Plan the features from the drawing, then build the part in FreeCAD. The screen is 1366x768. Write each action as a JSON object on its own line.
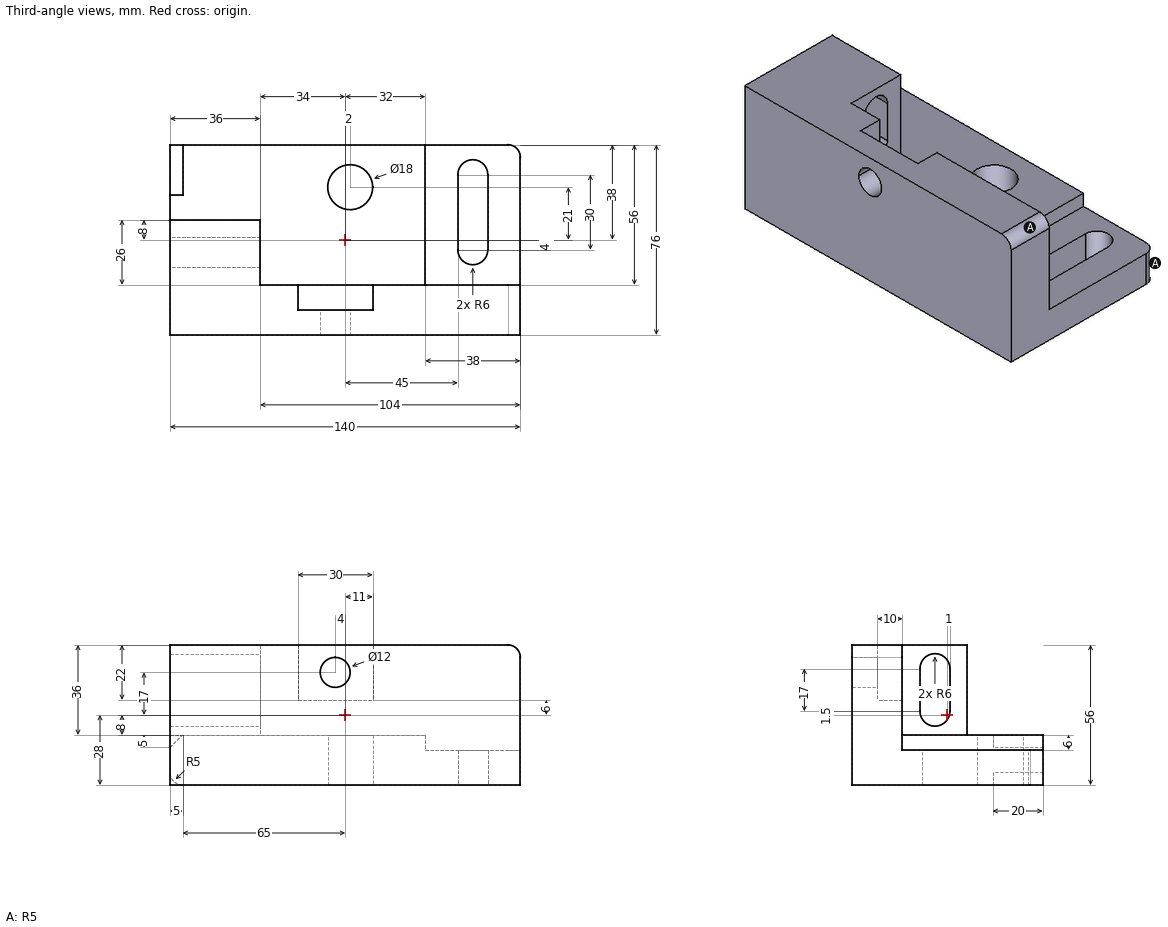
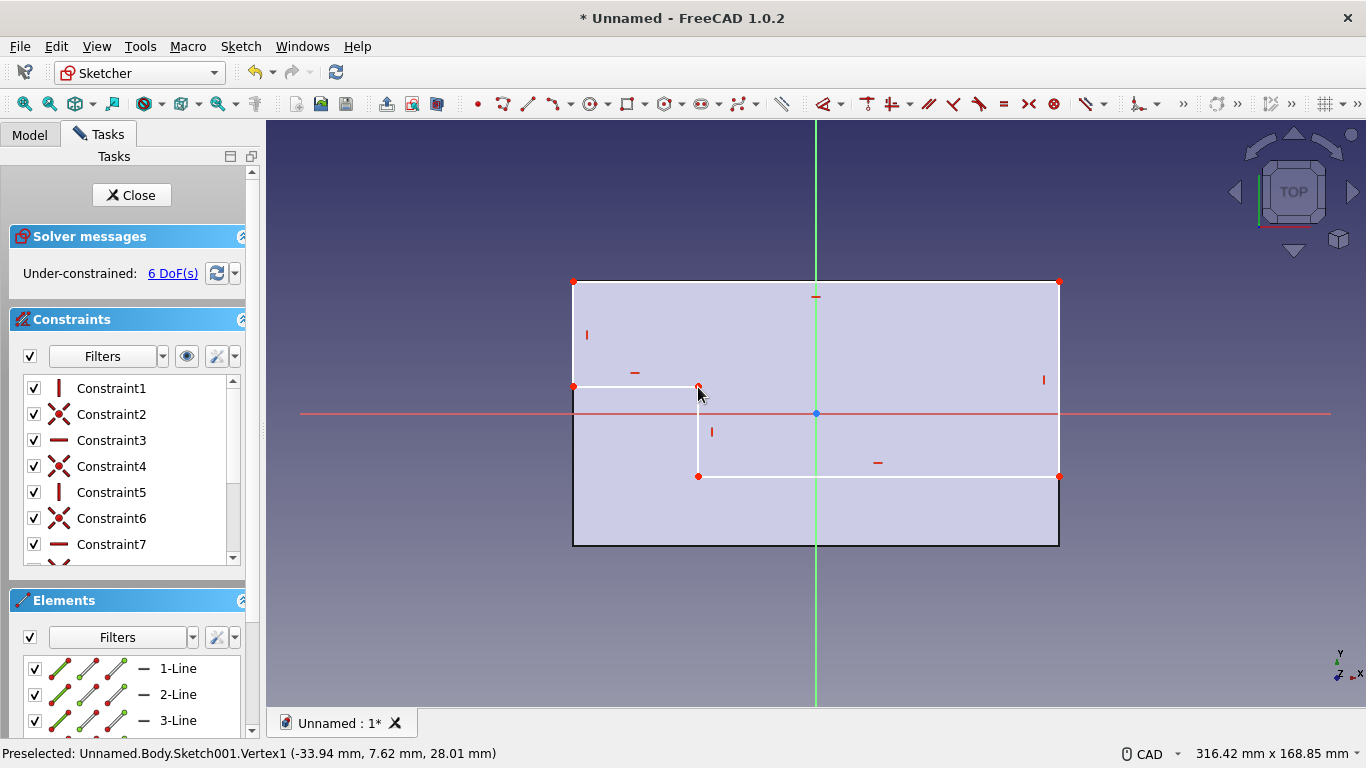
{"action": "left_click", "coordinate": [698, 414]}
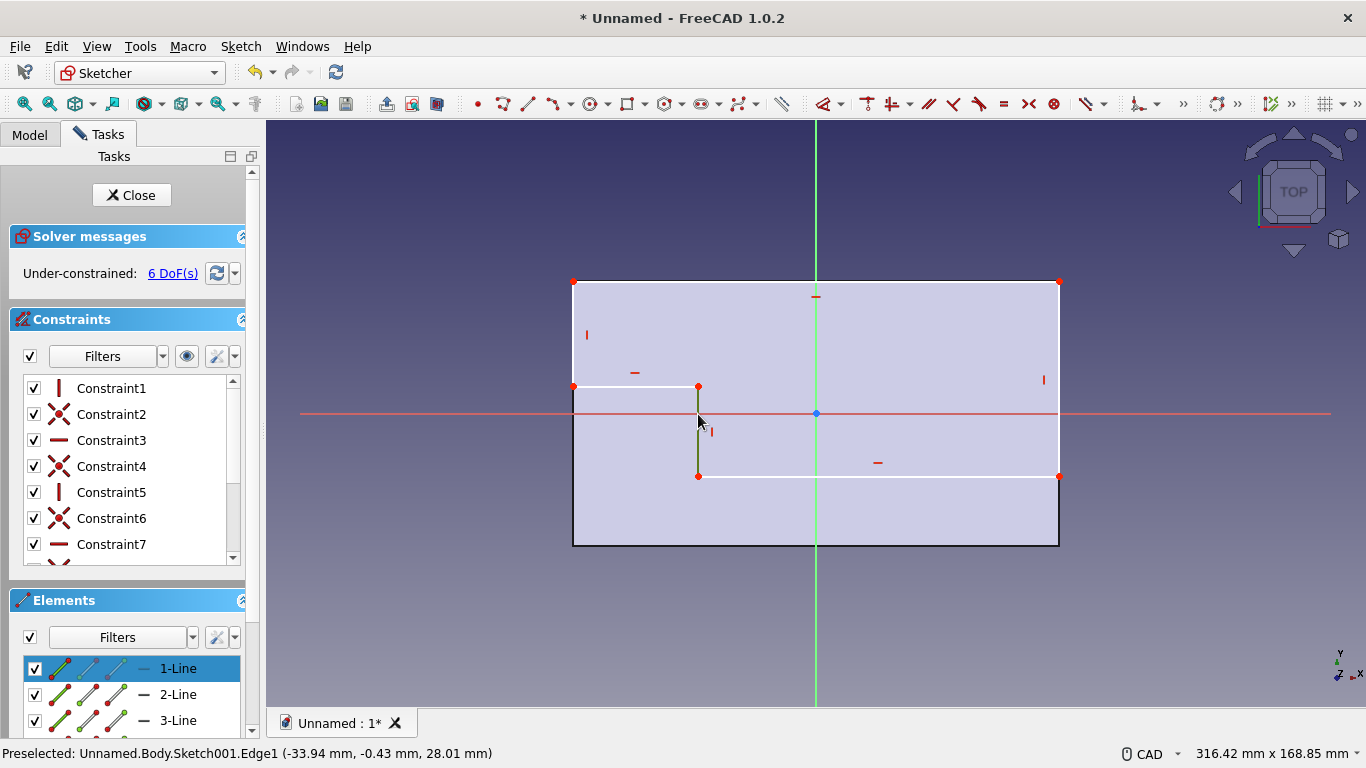
{"action": "key", "text": "i"}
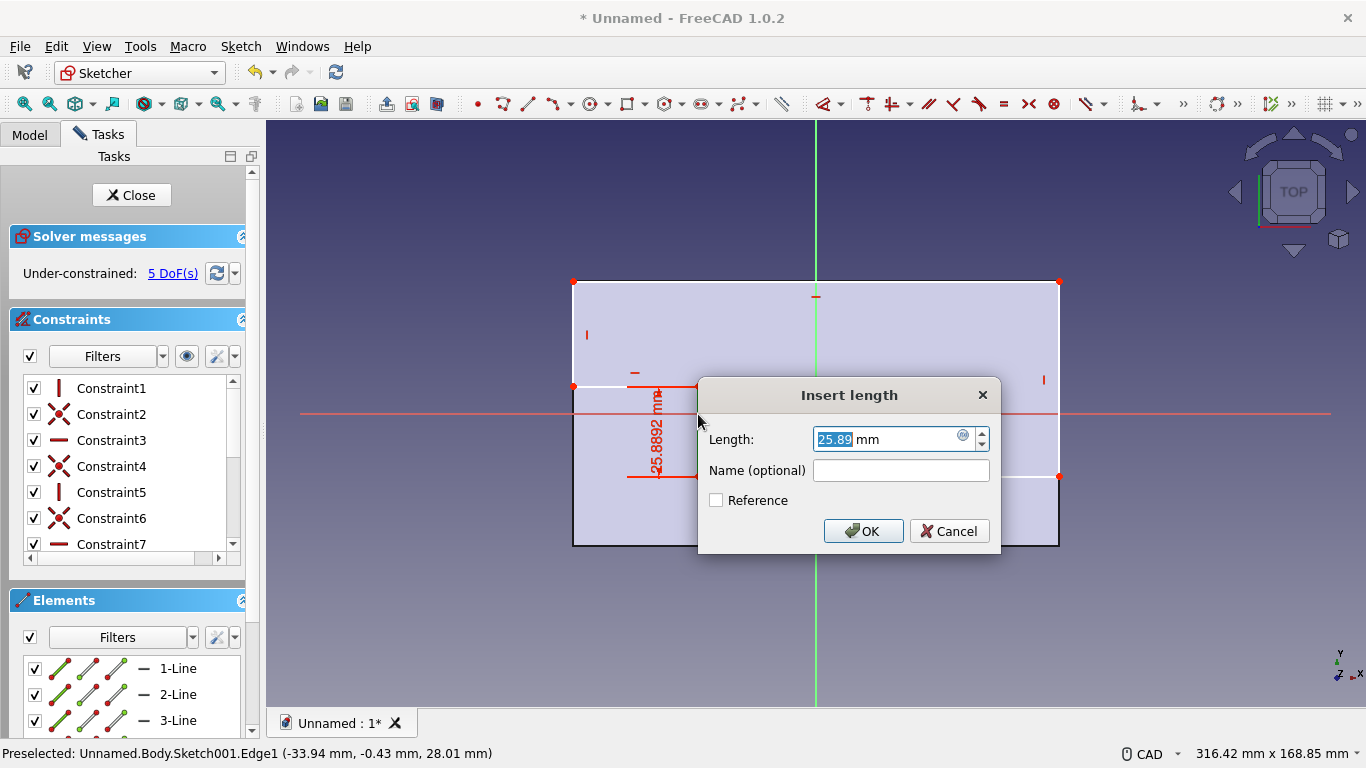
{"action": "type", "text": "26"}
{"action": "key", "text": "Return"}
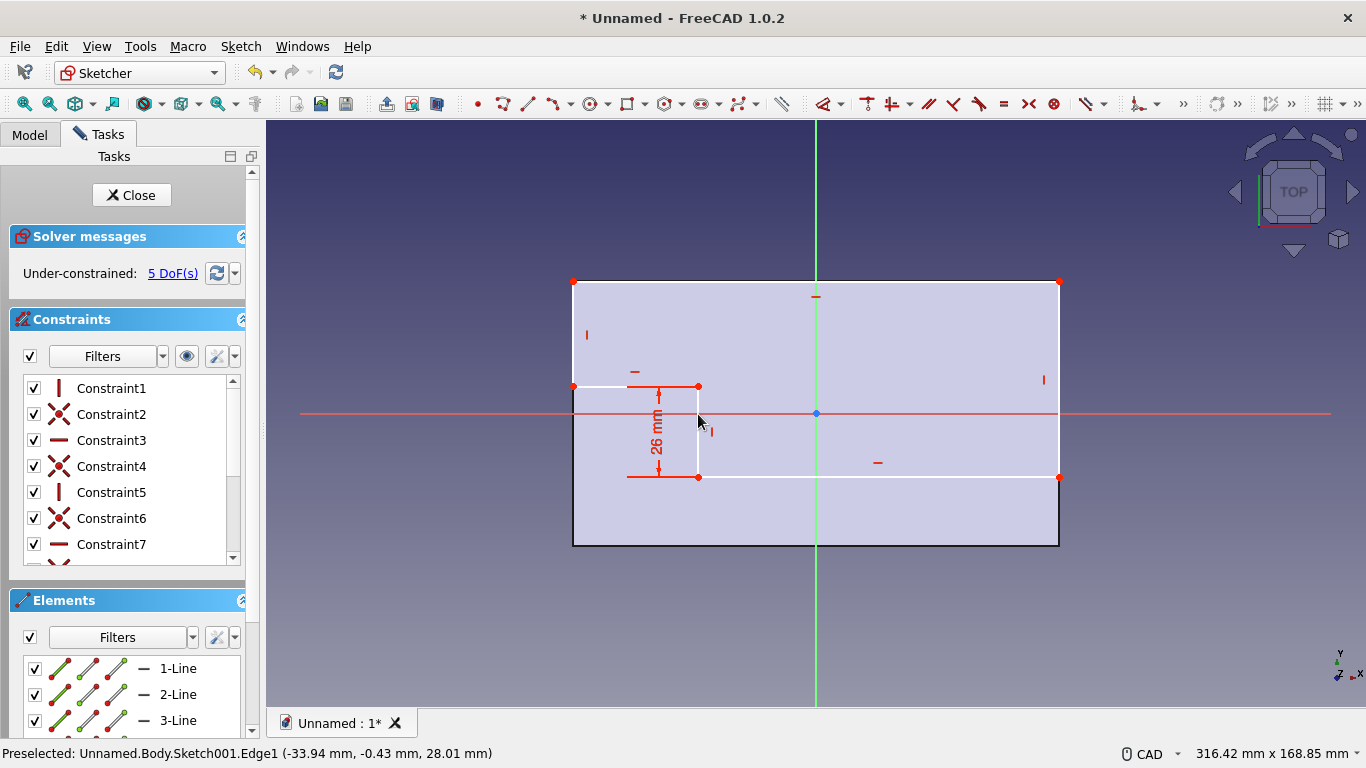
{"action": "left_click", "coordinate": [1059, 341]}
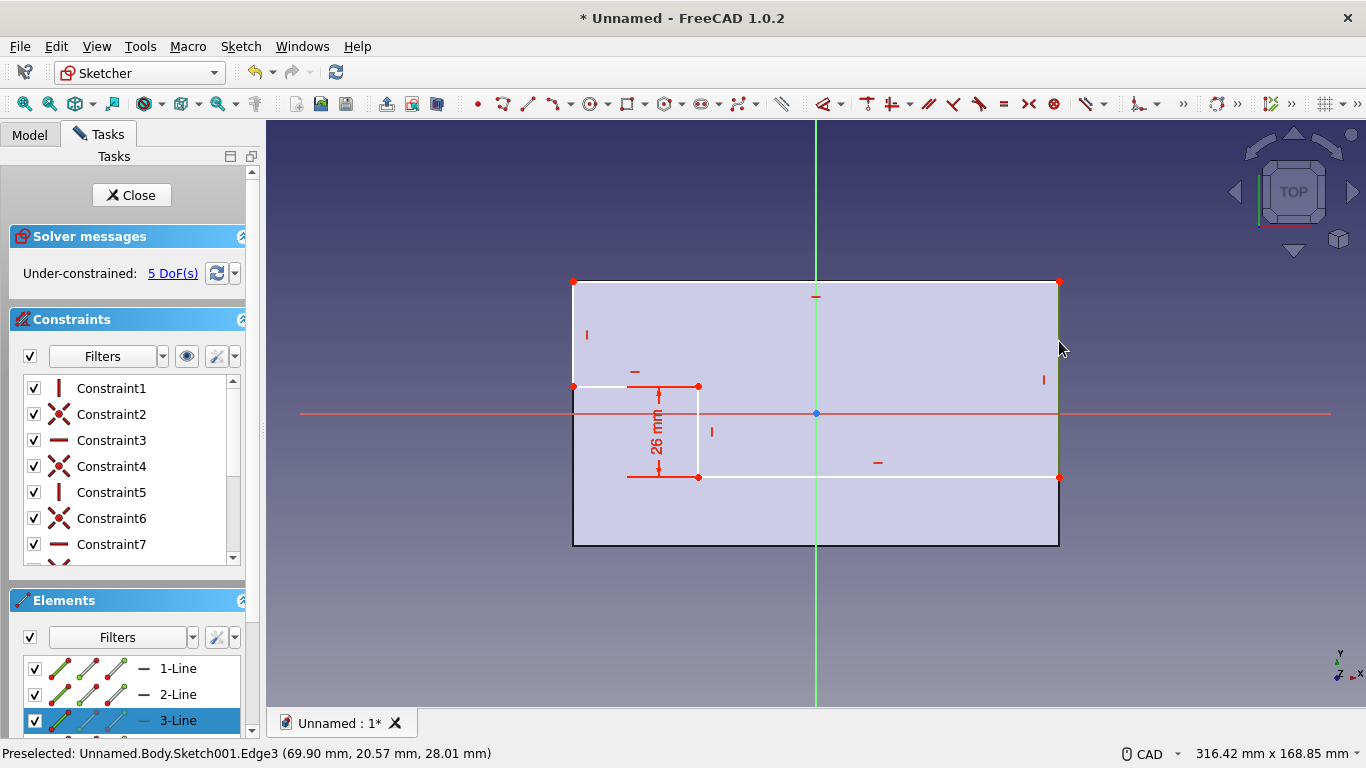
{"action": "left_click", "coordinate": [840, 104]}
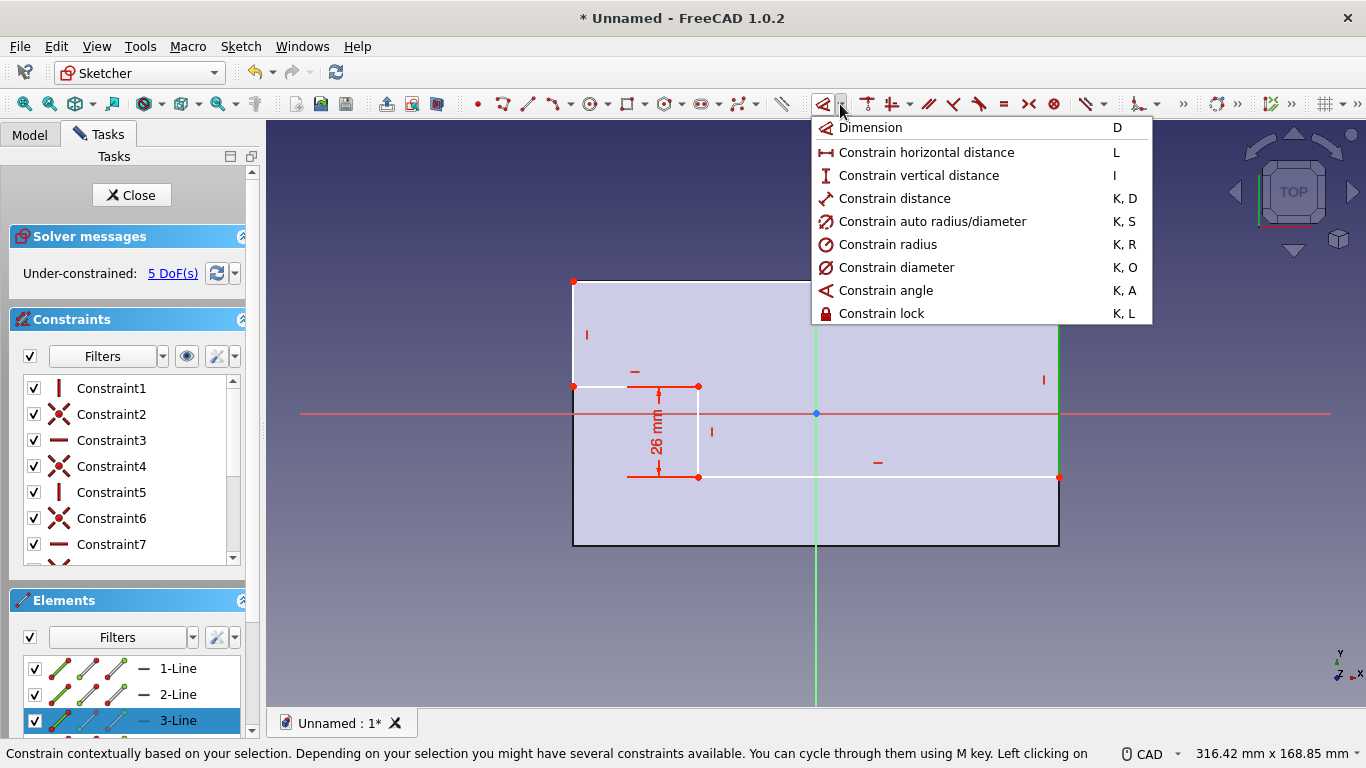
{"action": "left_click", "coordinate": [982, 176]}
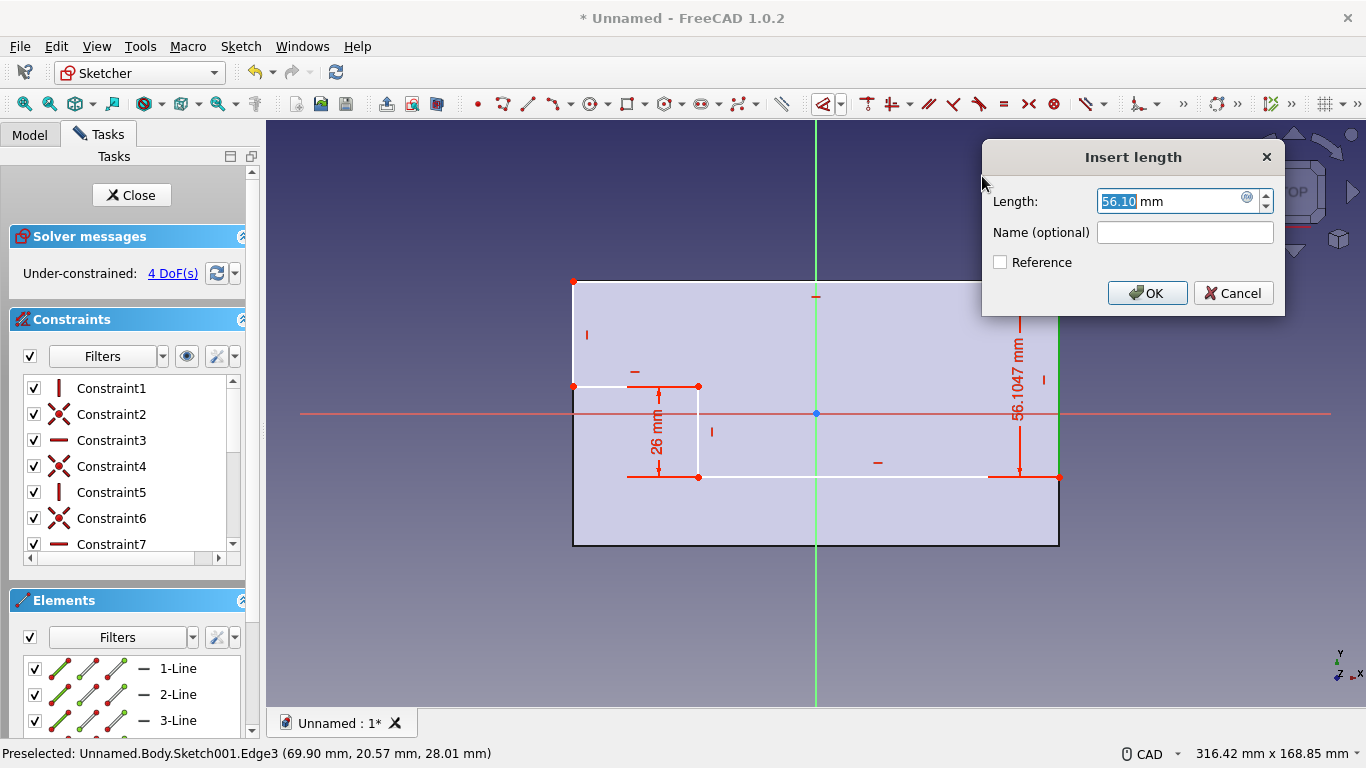
{"action": "type", "text": "56"}
{"action": "key", "text": "Return"}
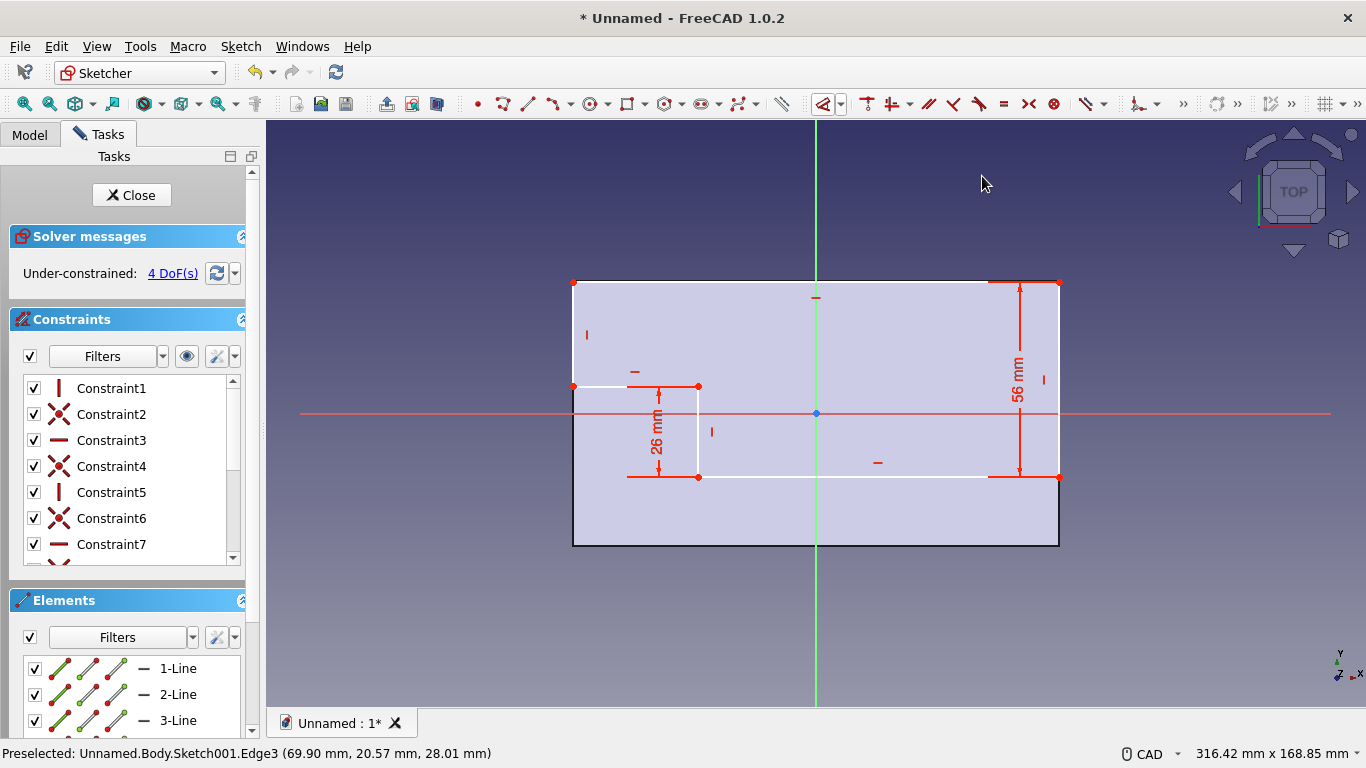
{"action": "left_click", "coordinate": [611, 387]}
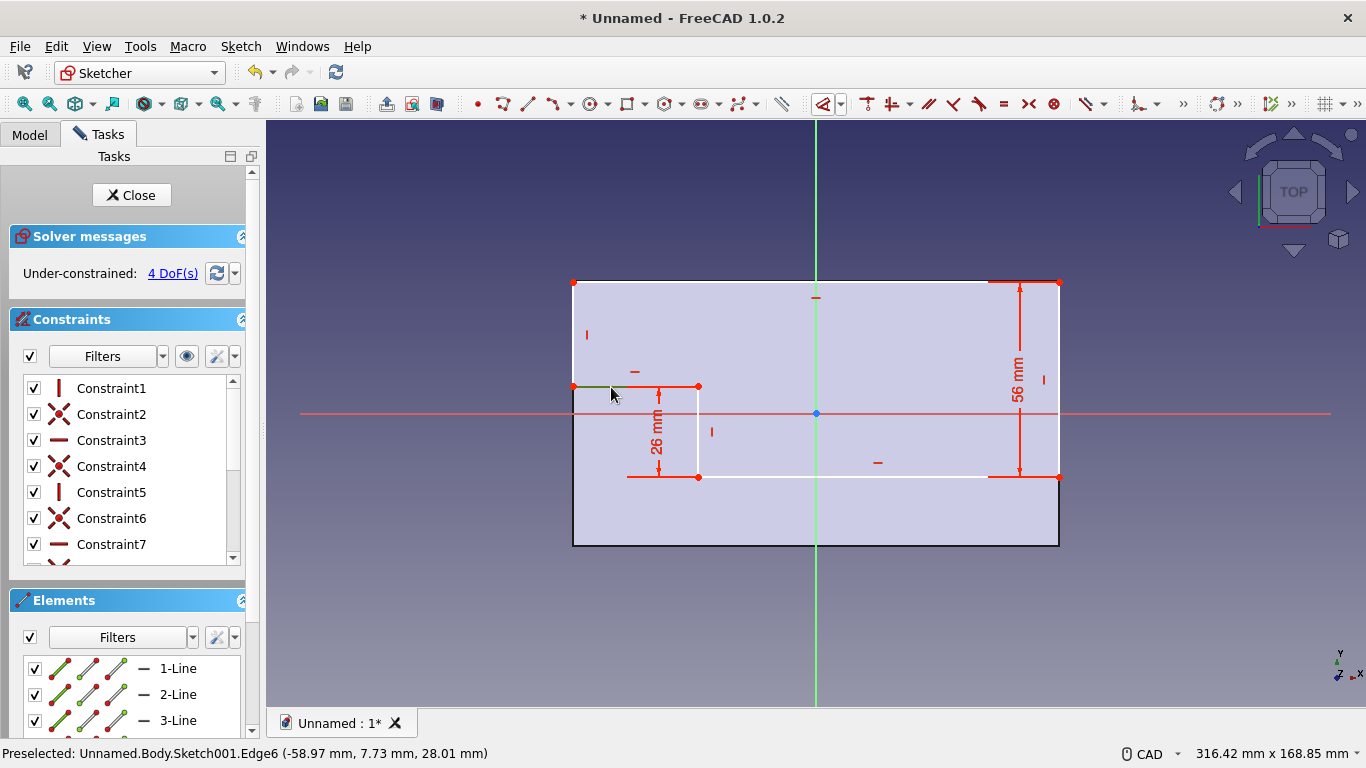
{"action": "key", "text": "l"}